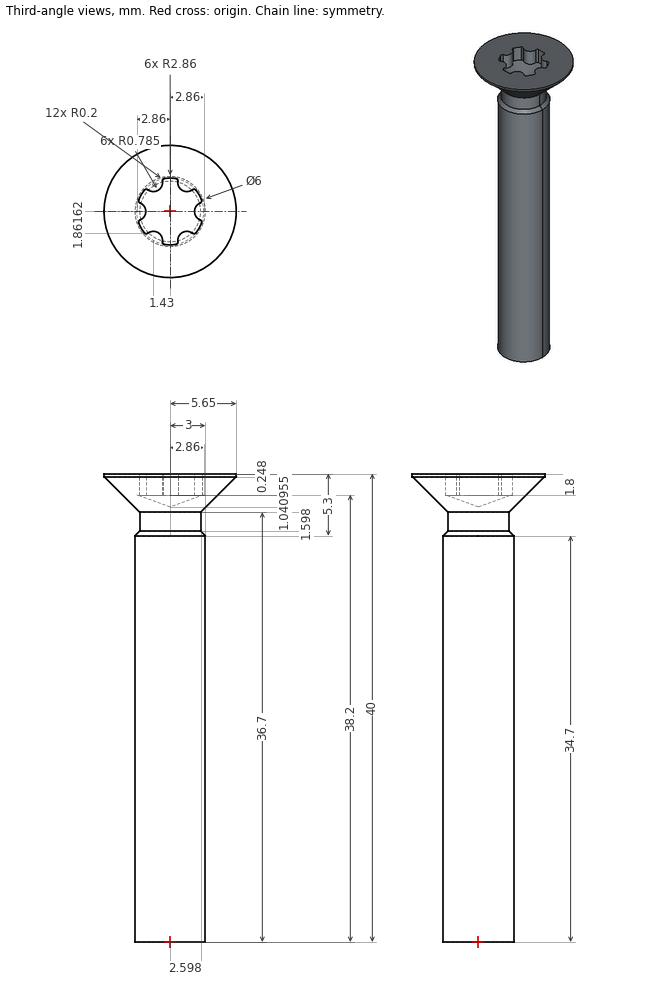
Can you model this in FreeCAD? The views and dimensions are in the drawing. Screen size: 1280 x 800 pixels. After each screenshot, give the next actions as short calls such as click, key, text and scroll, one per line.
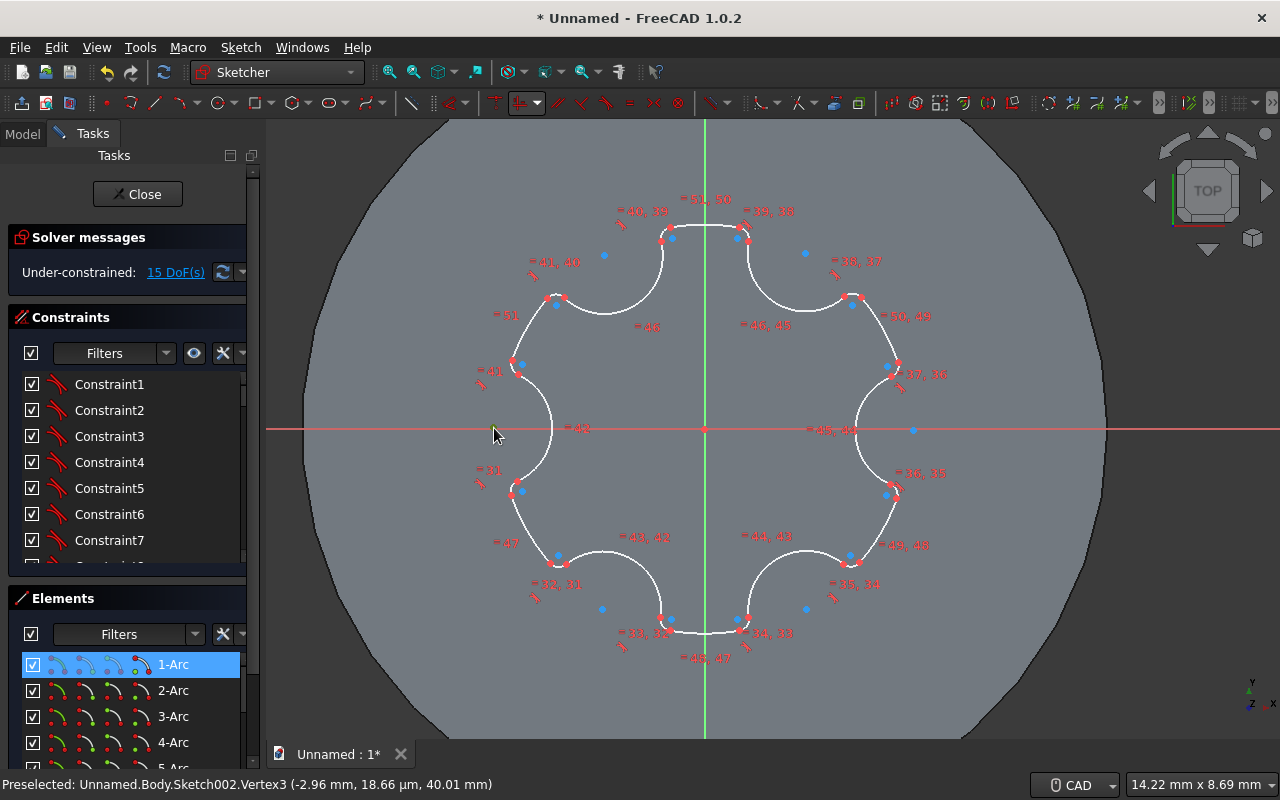
click(353, 429)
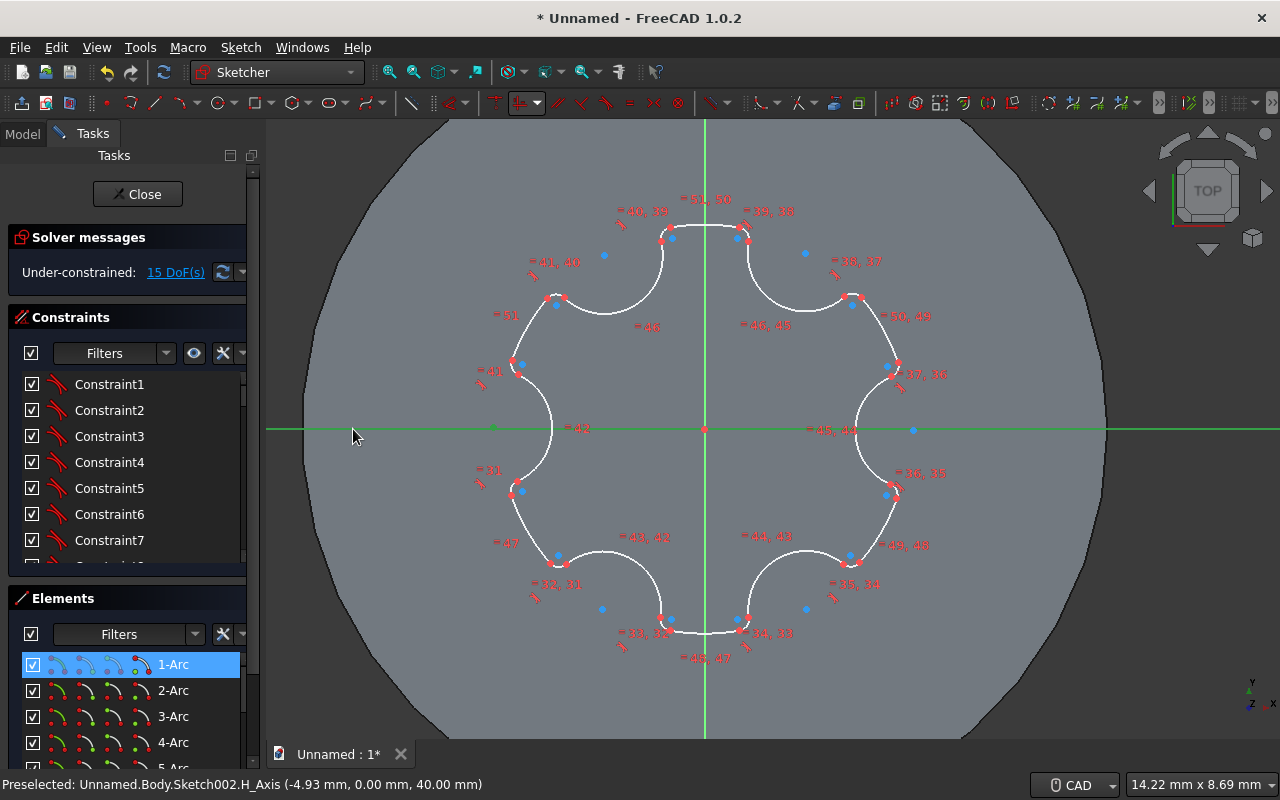
click(496, 104)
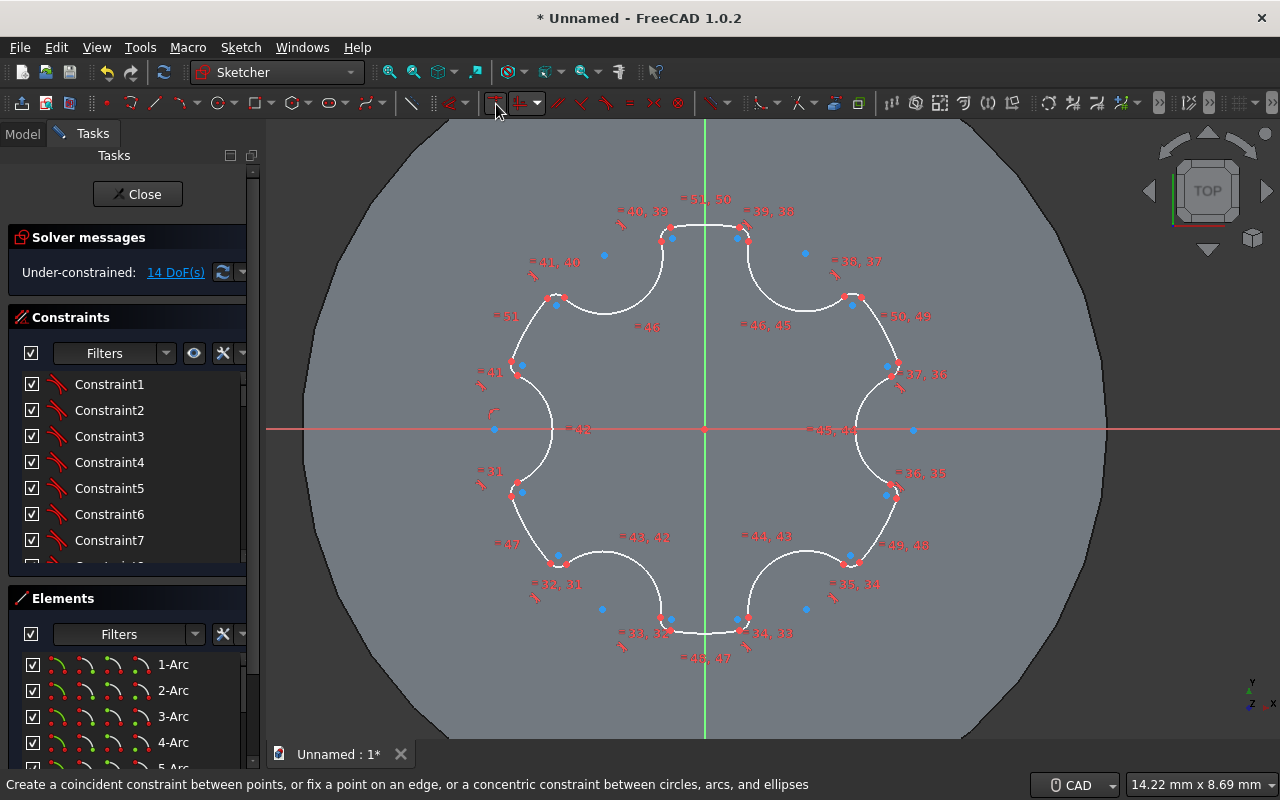
click(914, 431)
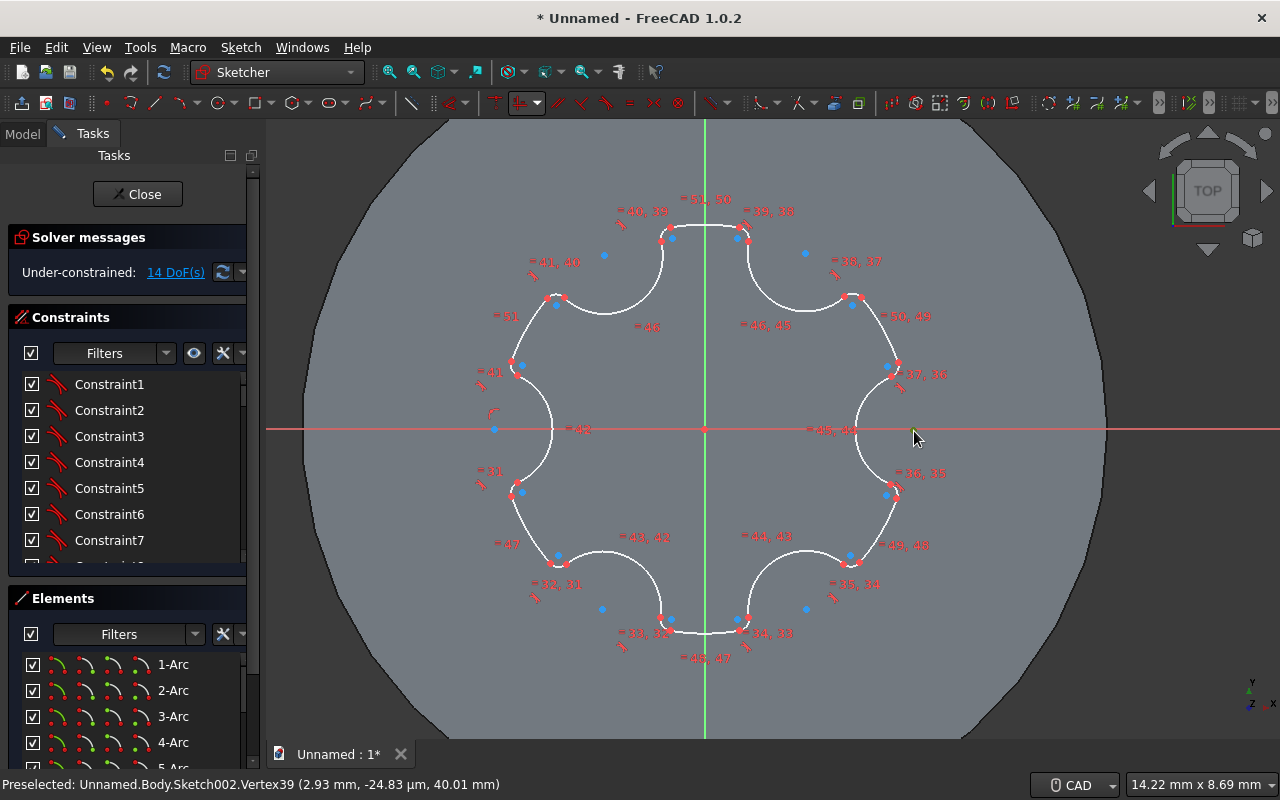
click(353, 429)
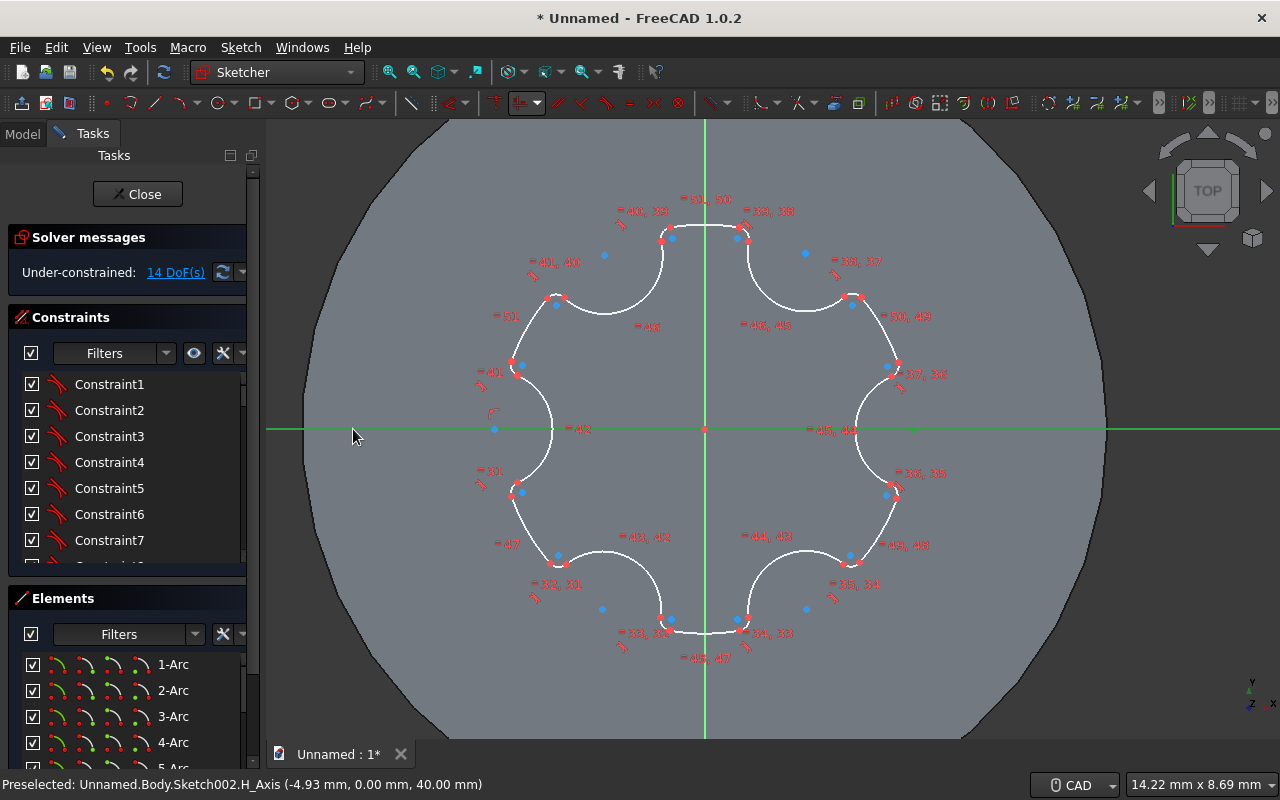
click(496, 104)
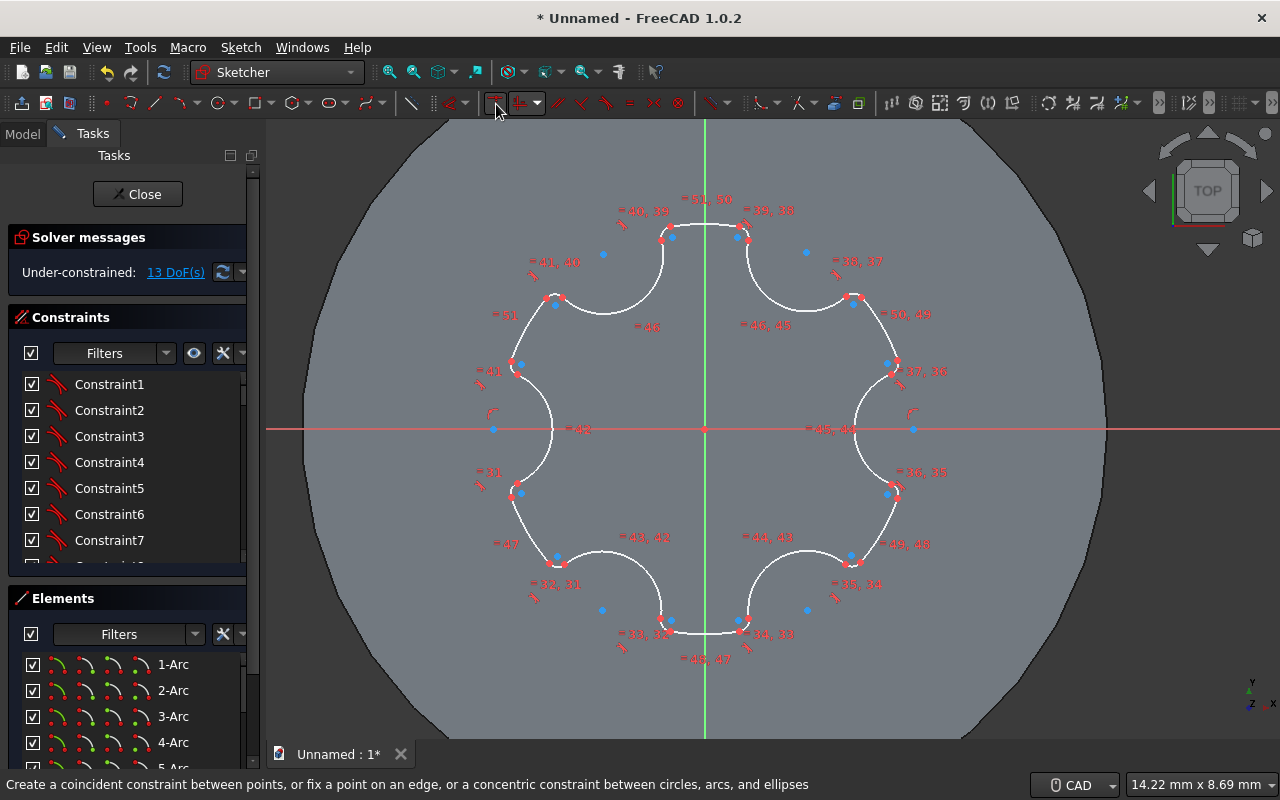
click(602, 611)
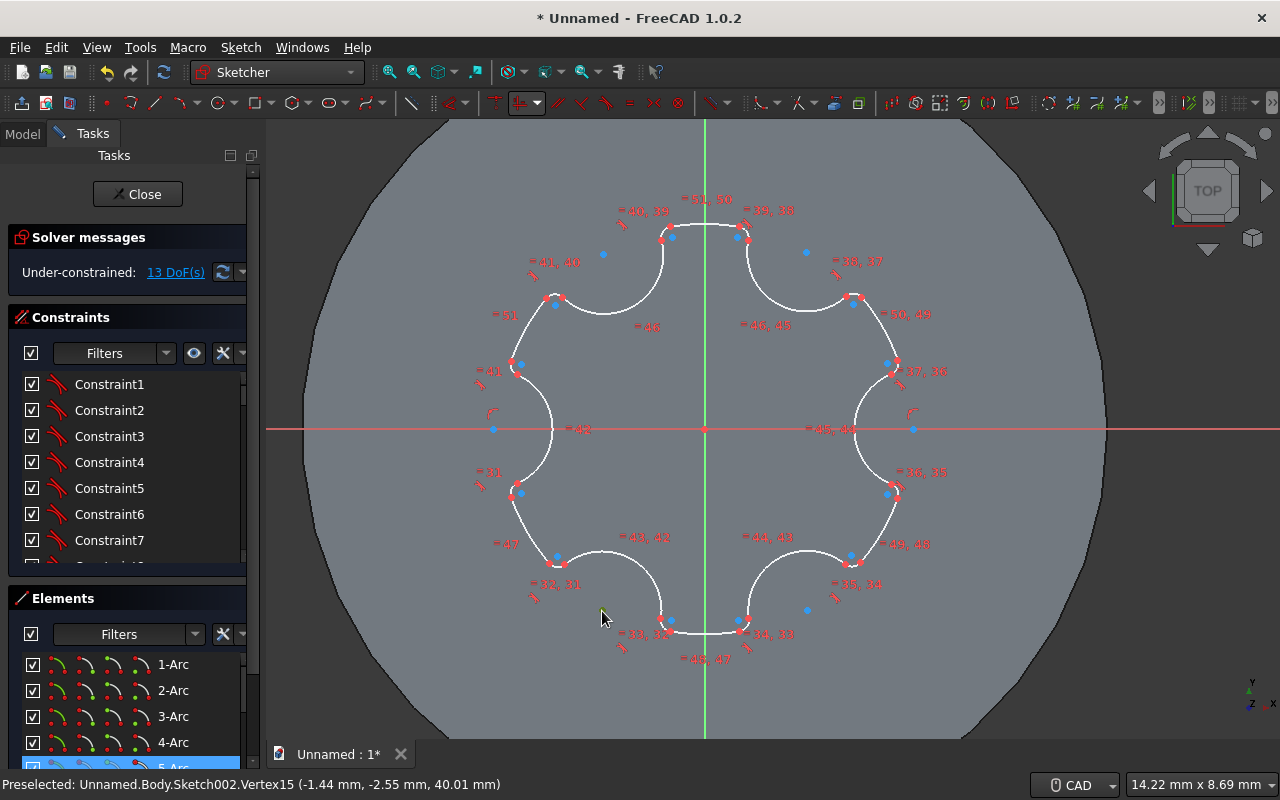
click(808, 610)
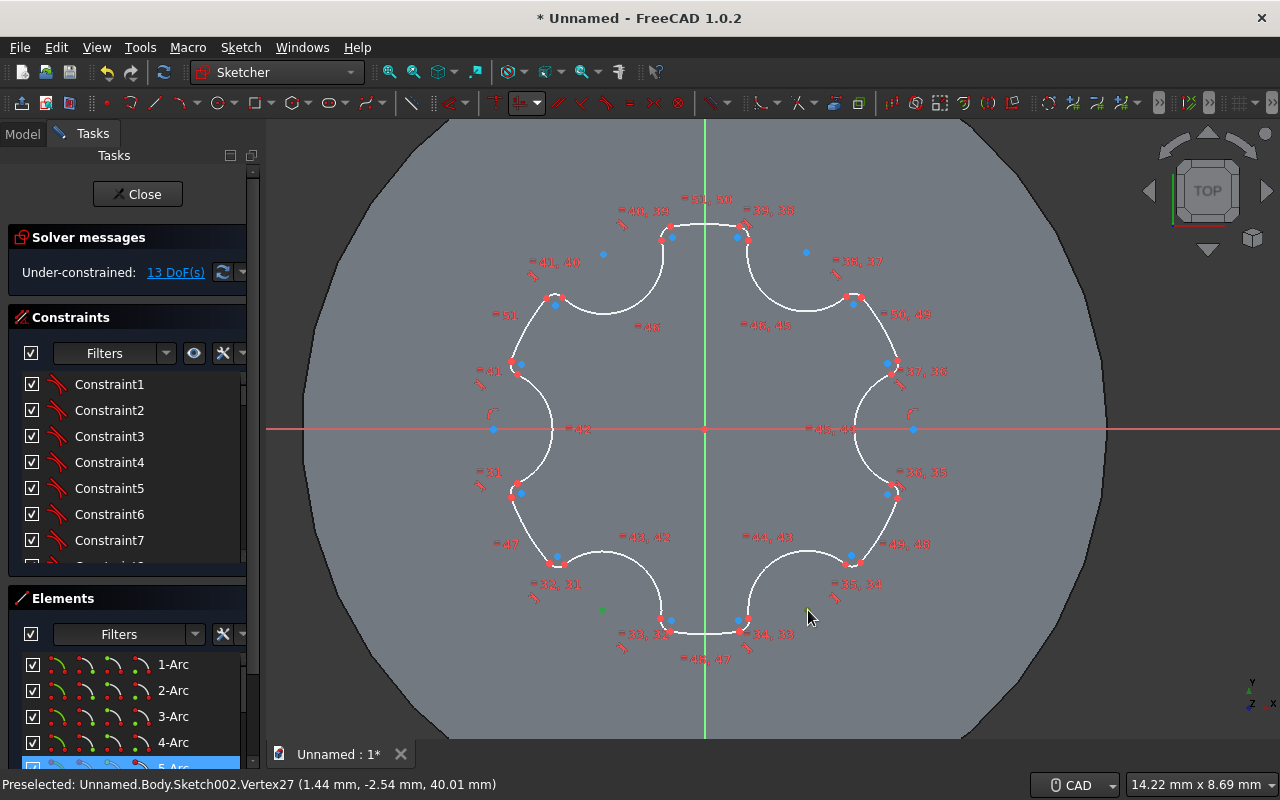
click(705, 671)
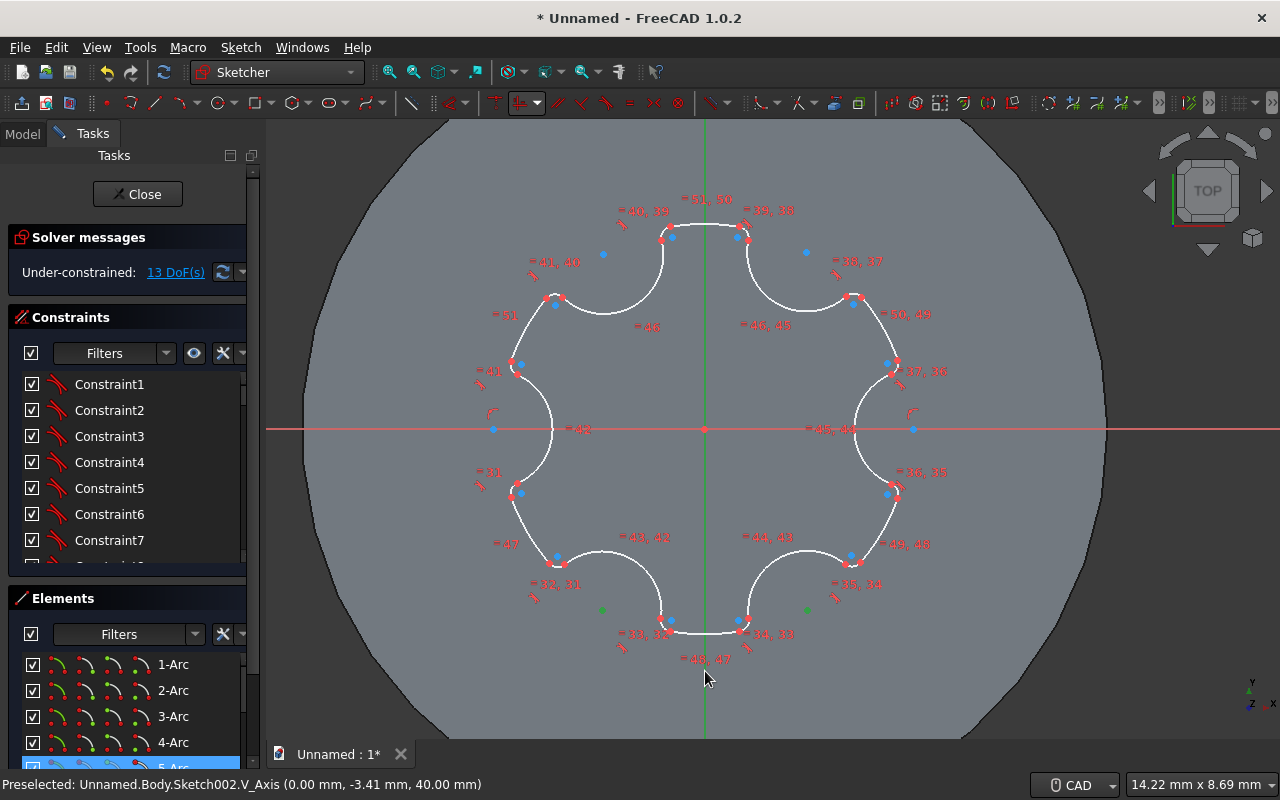
click(654, 104)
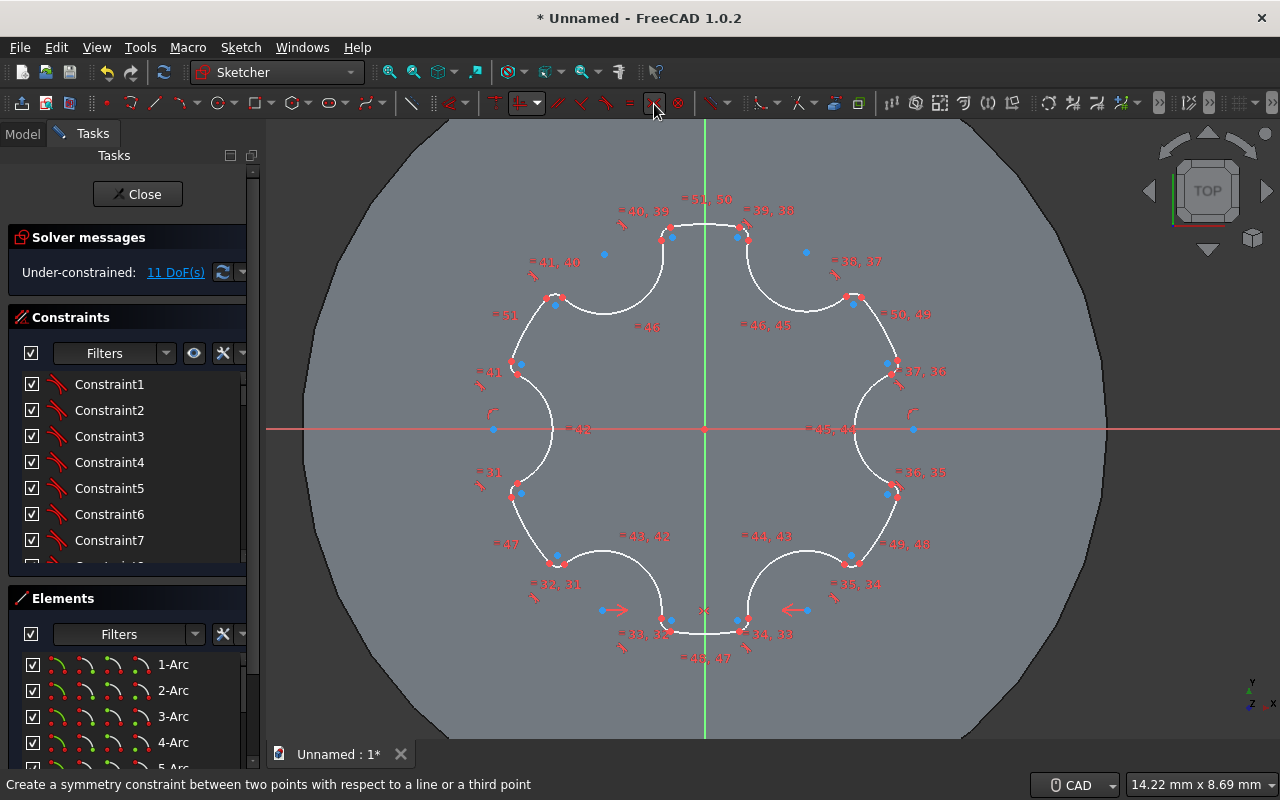
click(807, 610)